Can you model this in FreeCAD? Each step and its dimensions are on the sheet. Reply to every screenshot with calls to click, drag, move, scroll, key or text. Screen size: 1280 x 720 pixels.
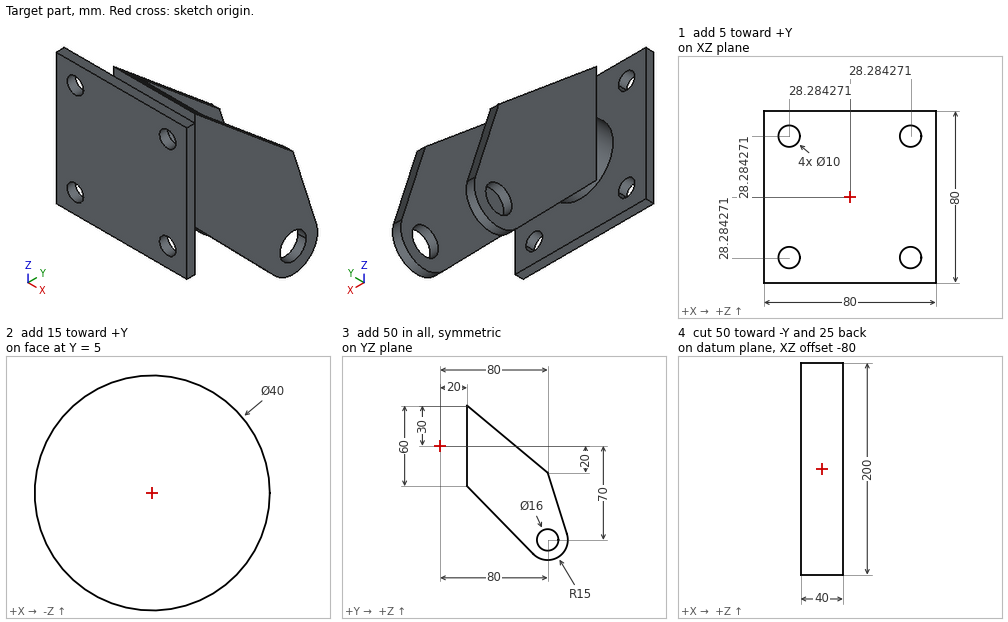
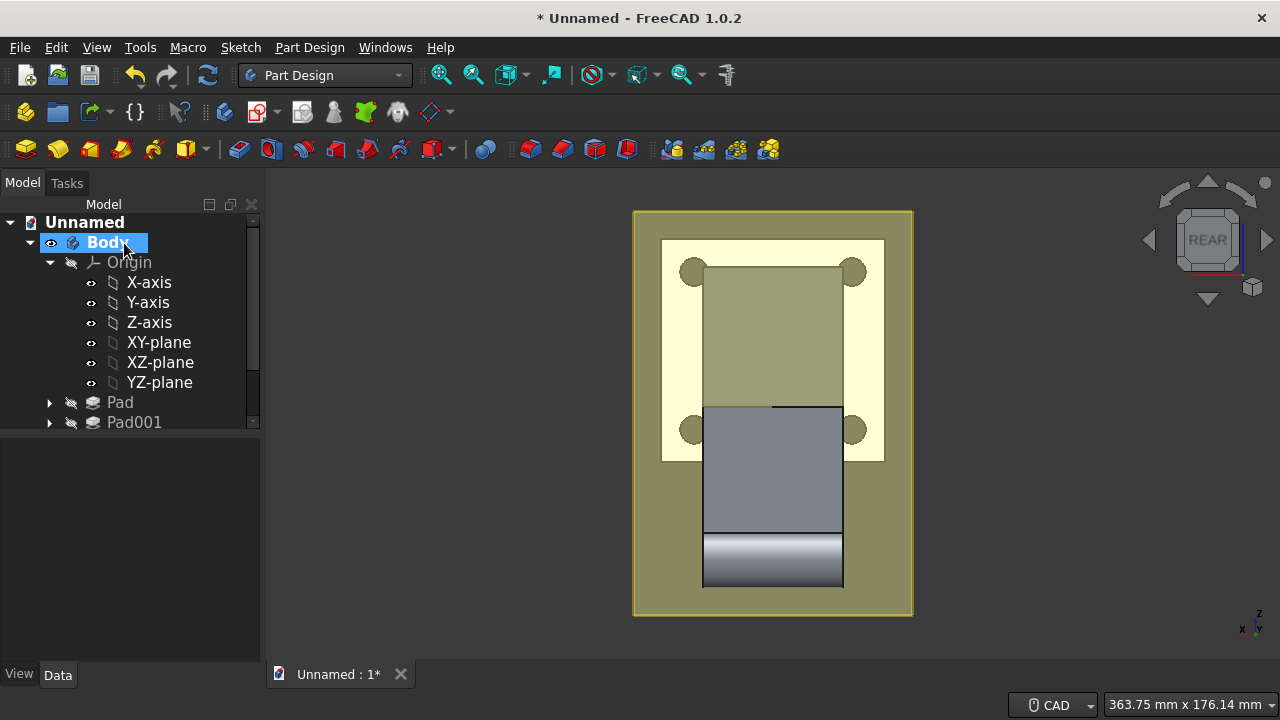
scroll(100, 318, down, 3)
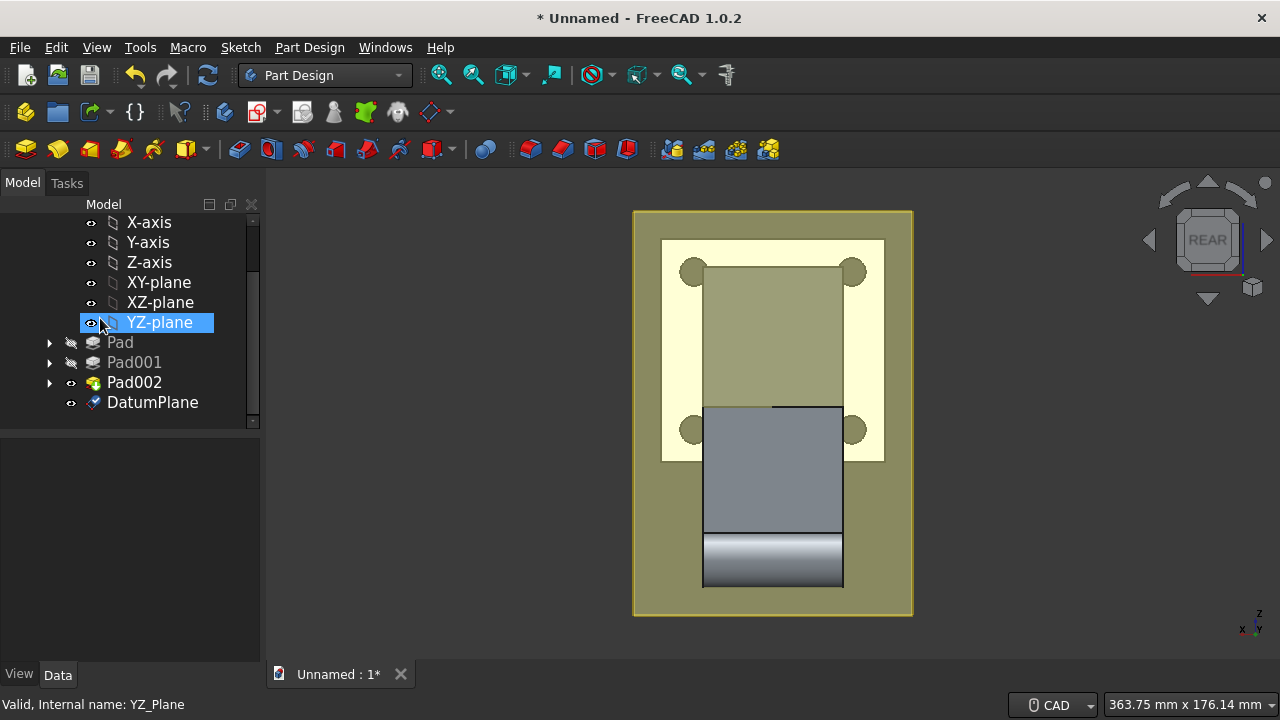
click(116, 403)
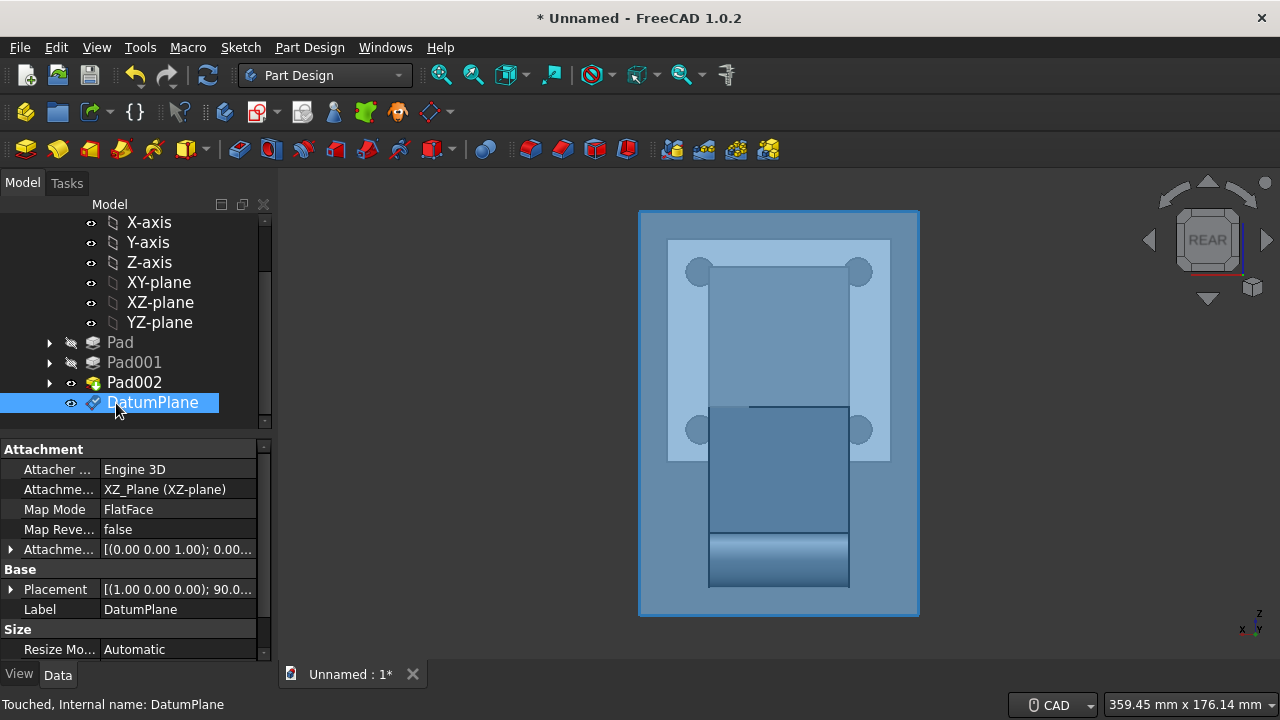
click(258, 112)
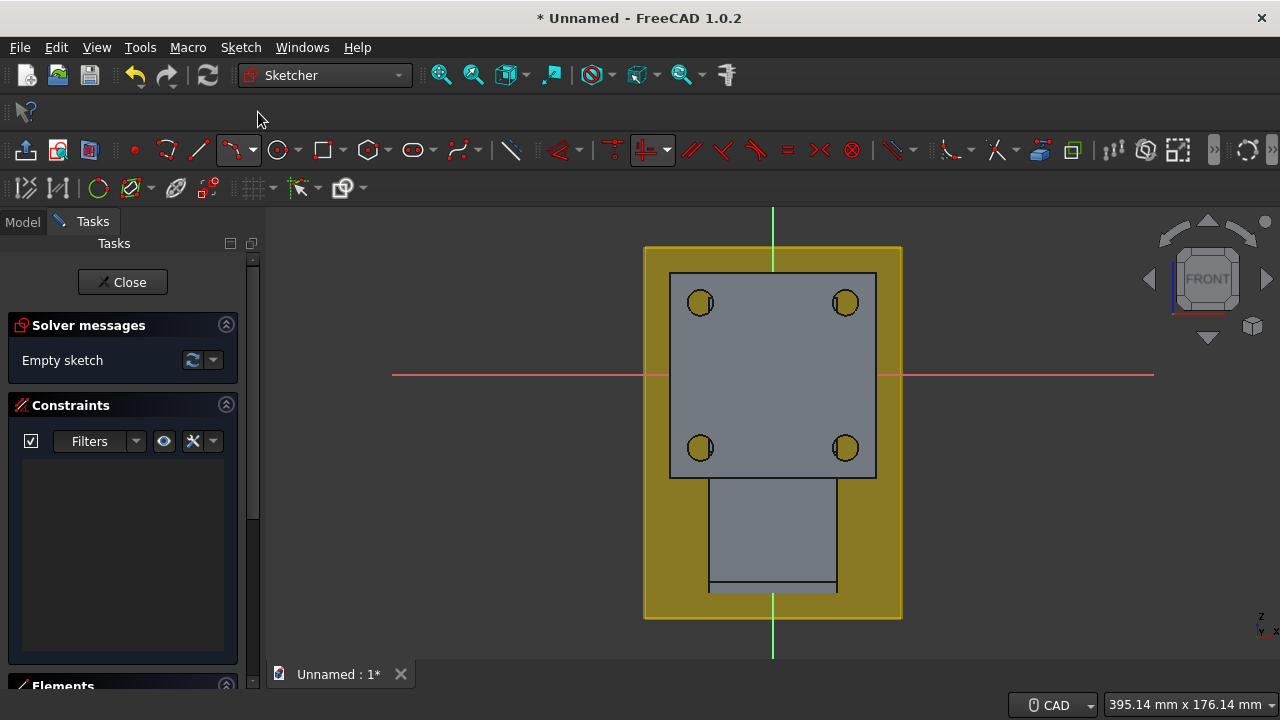
click(90, 150)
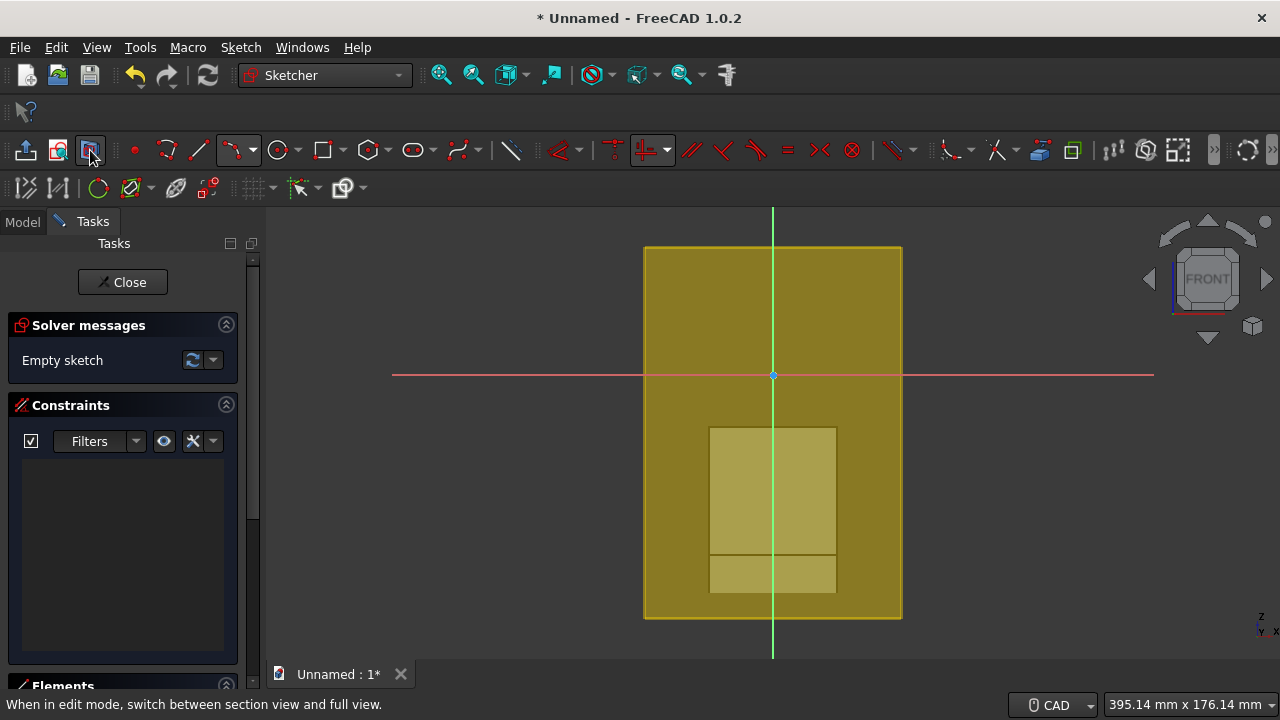
scroll(621, 503, down, 3)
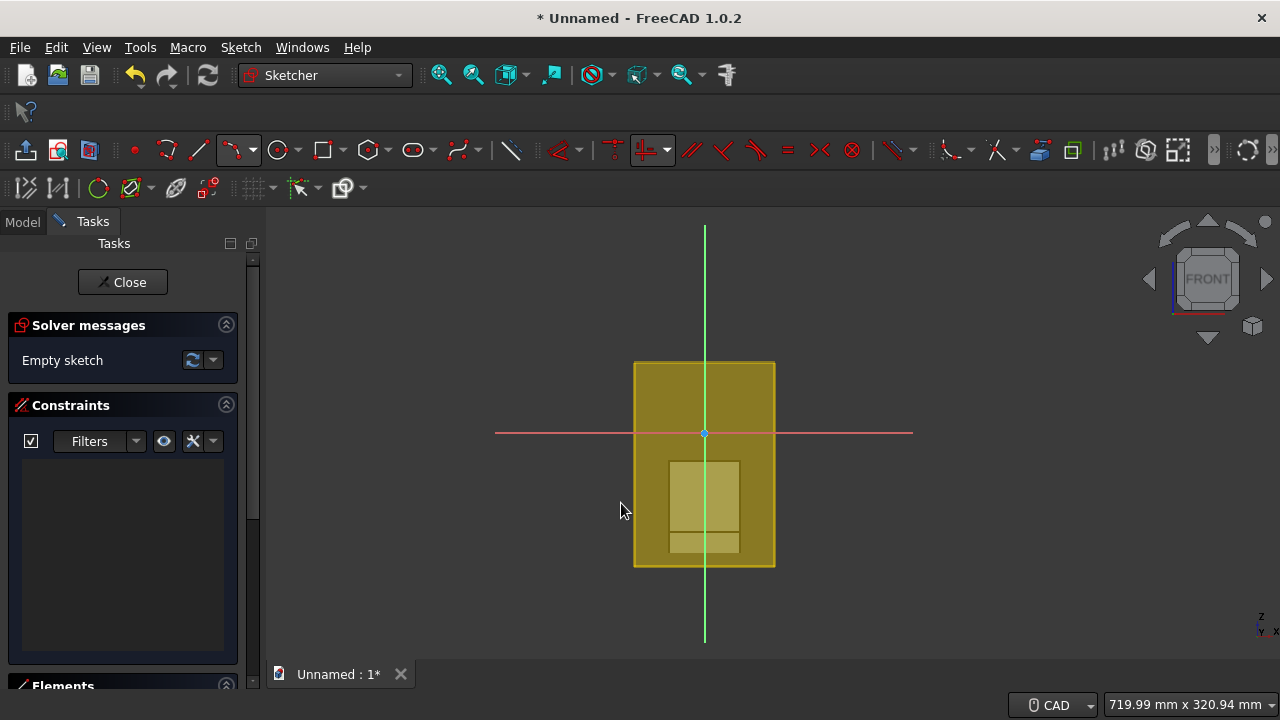
click(346, 150)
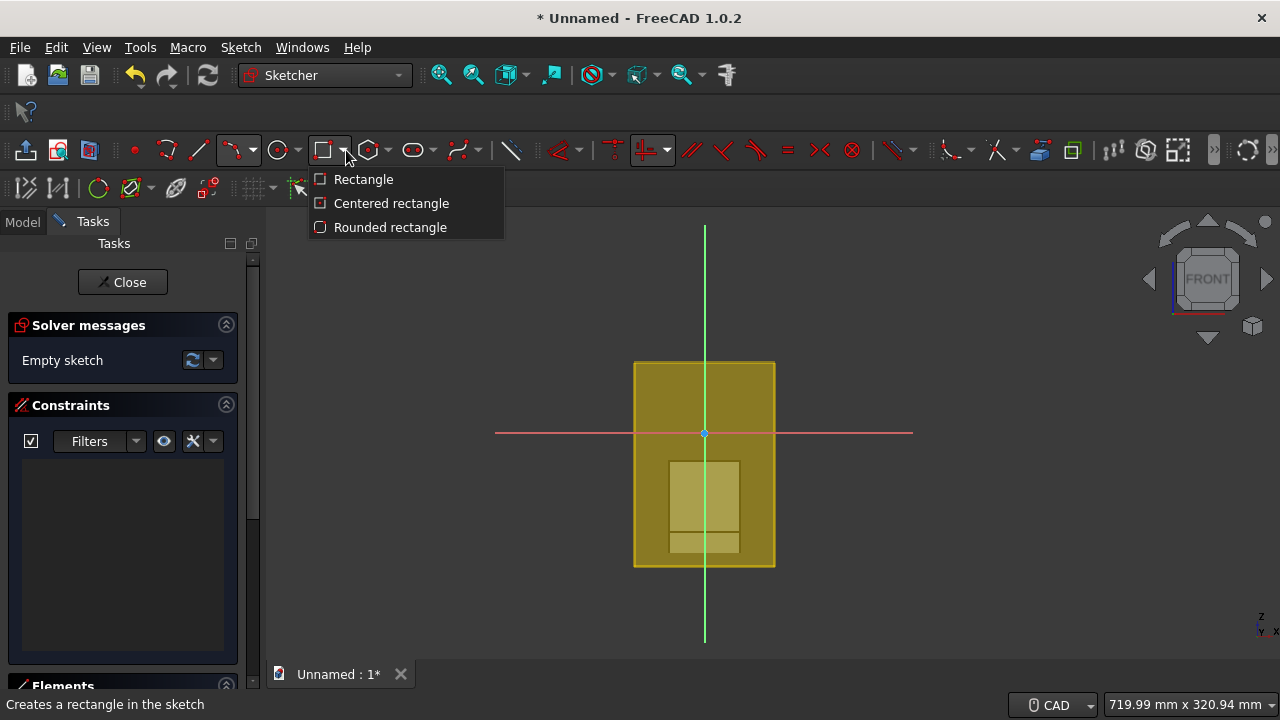
click(406, 203)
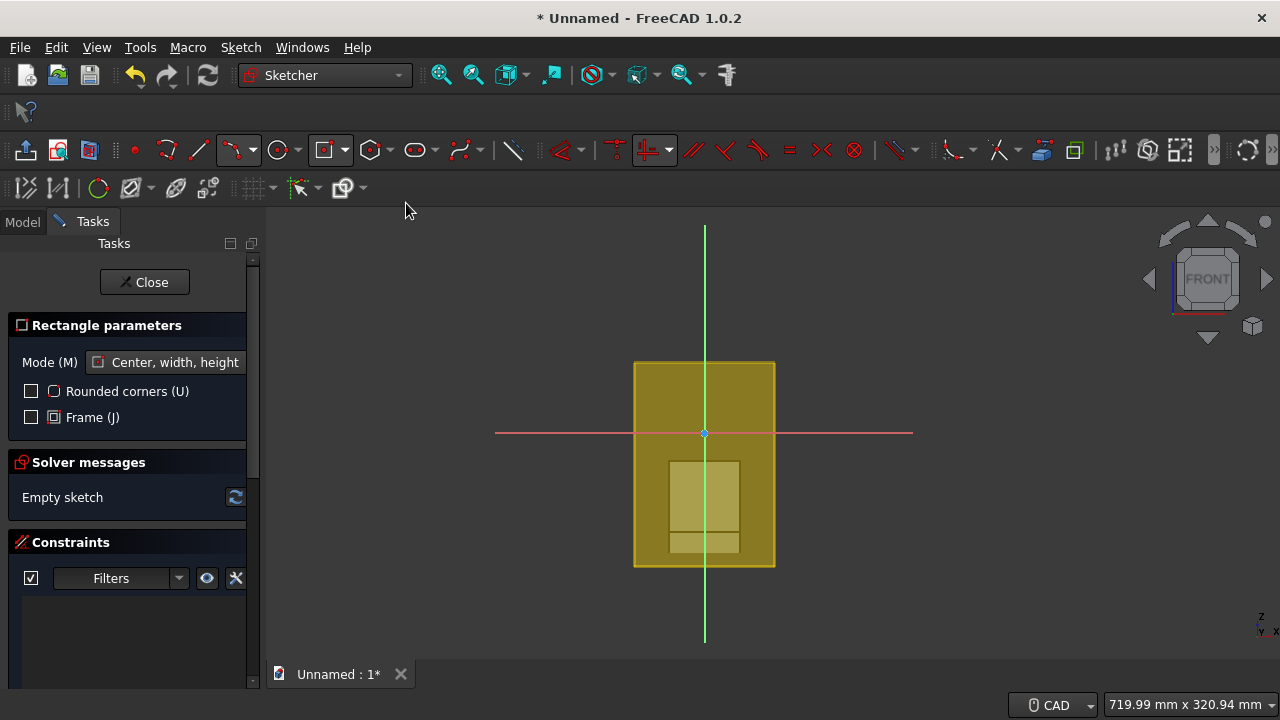
click(705, 433)
click(733, 292)
key(Escape)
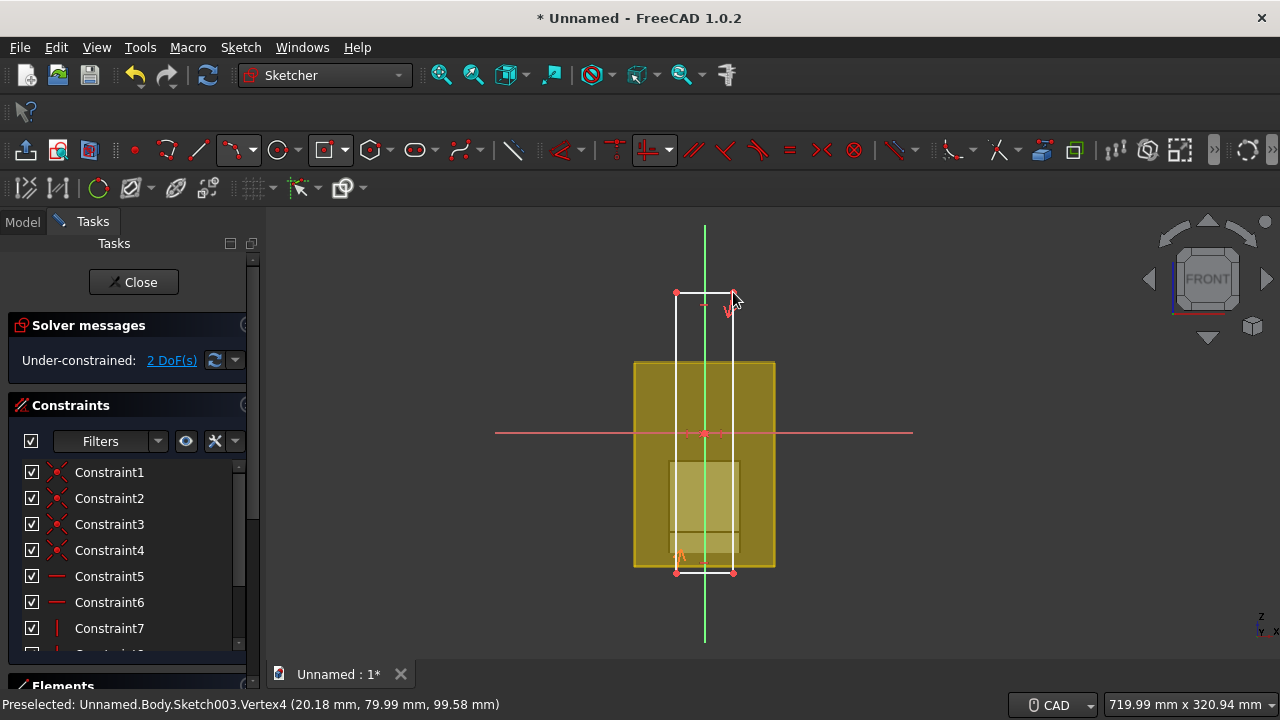
click(560, 150)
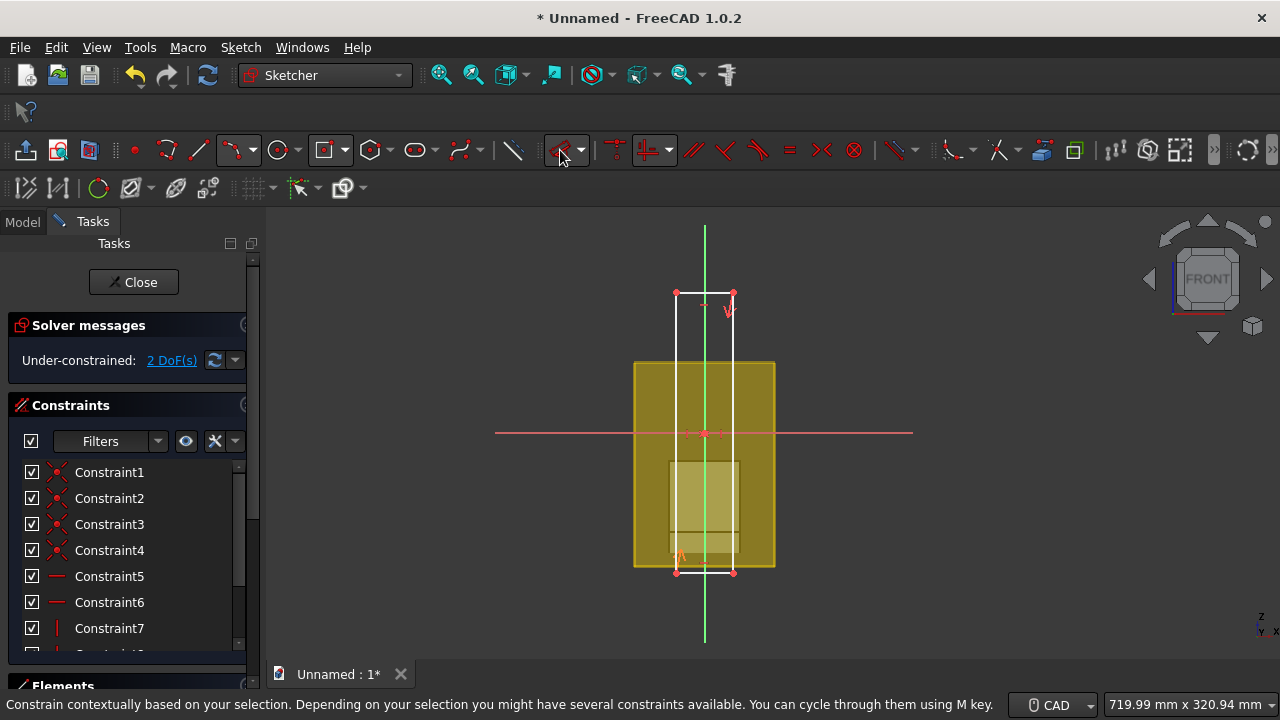
click(693, 573)
click(692, 607)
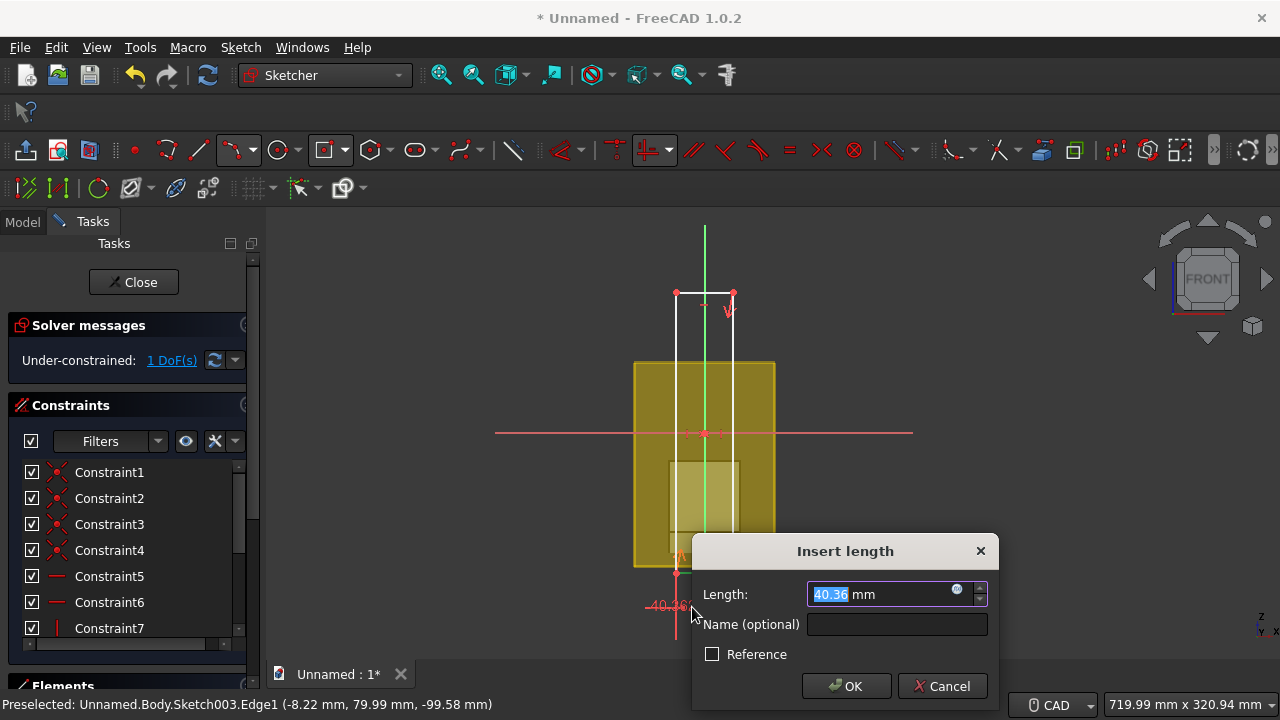
text(40)
key(Return)